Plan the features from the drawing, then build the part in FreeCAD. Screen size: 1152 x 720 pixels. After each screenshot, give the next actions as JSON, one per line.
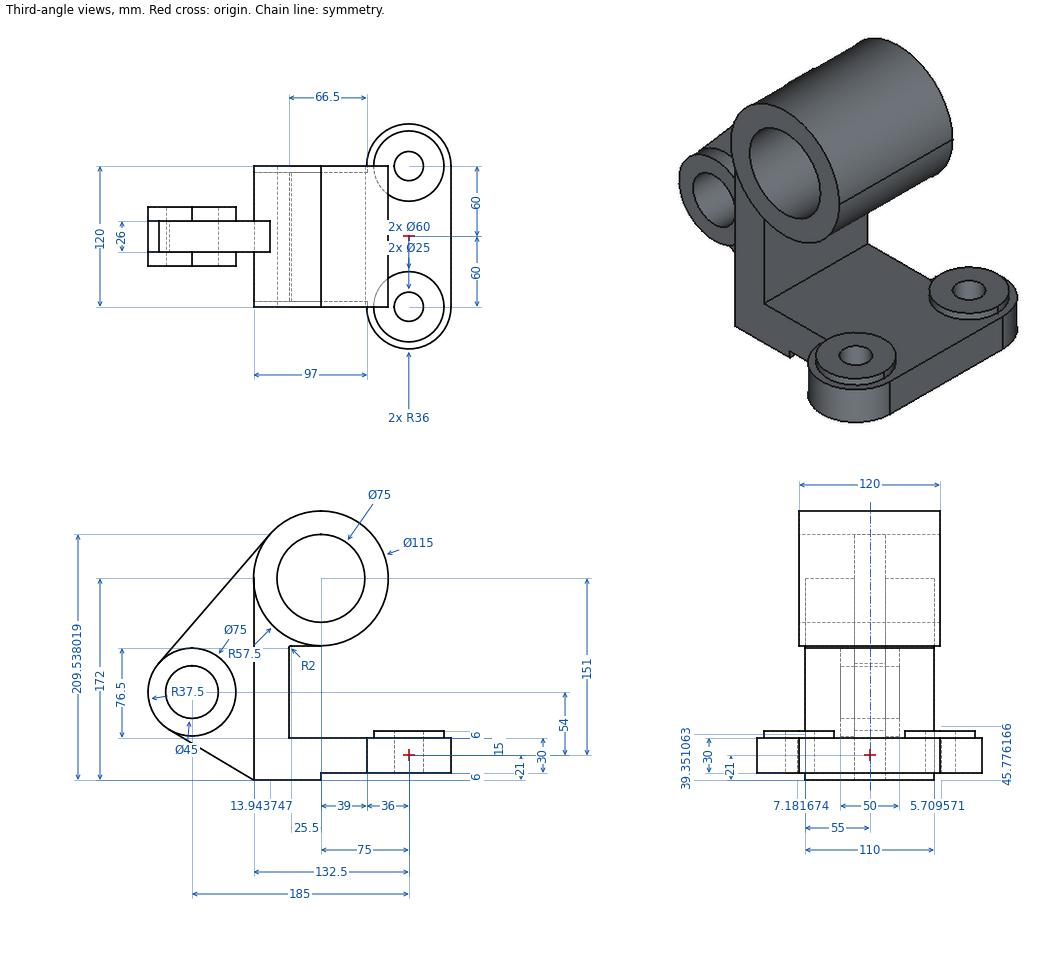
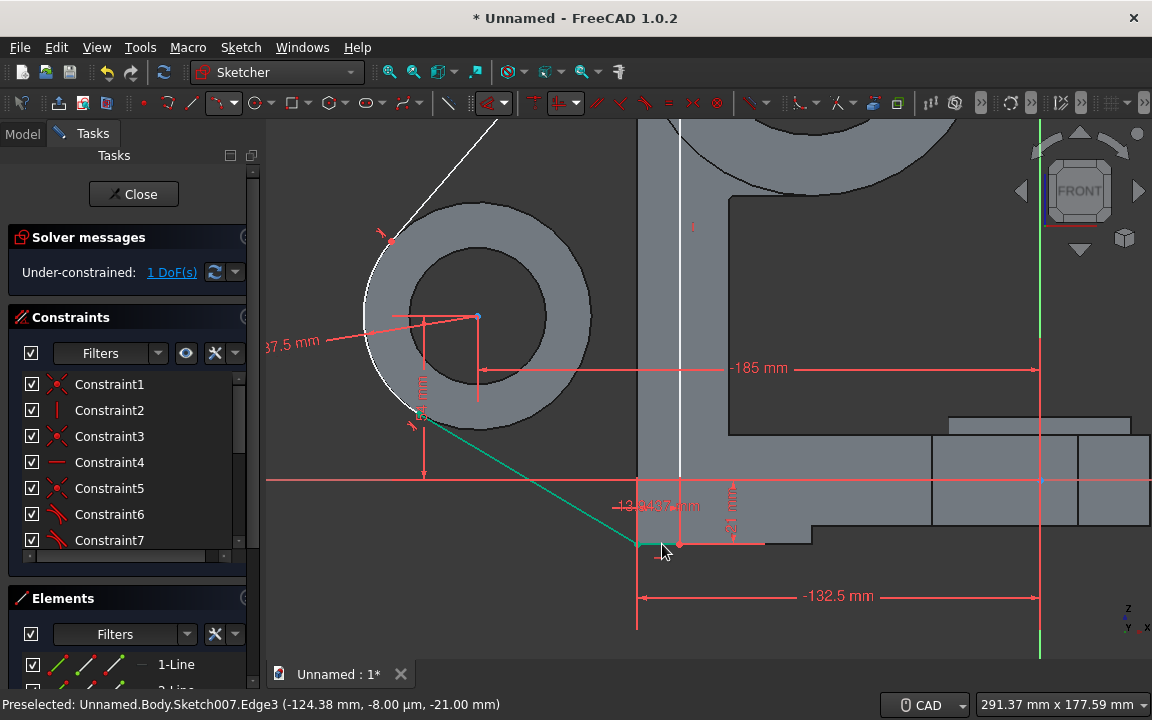
{"action": "left_click", "coordinate": [680, 353]}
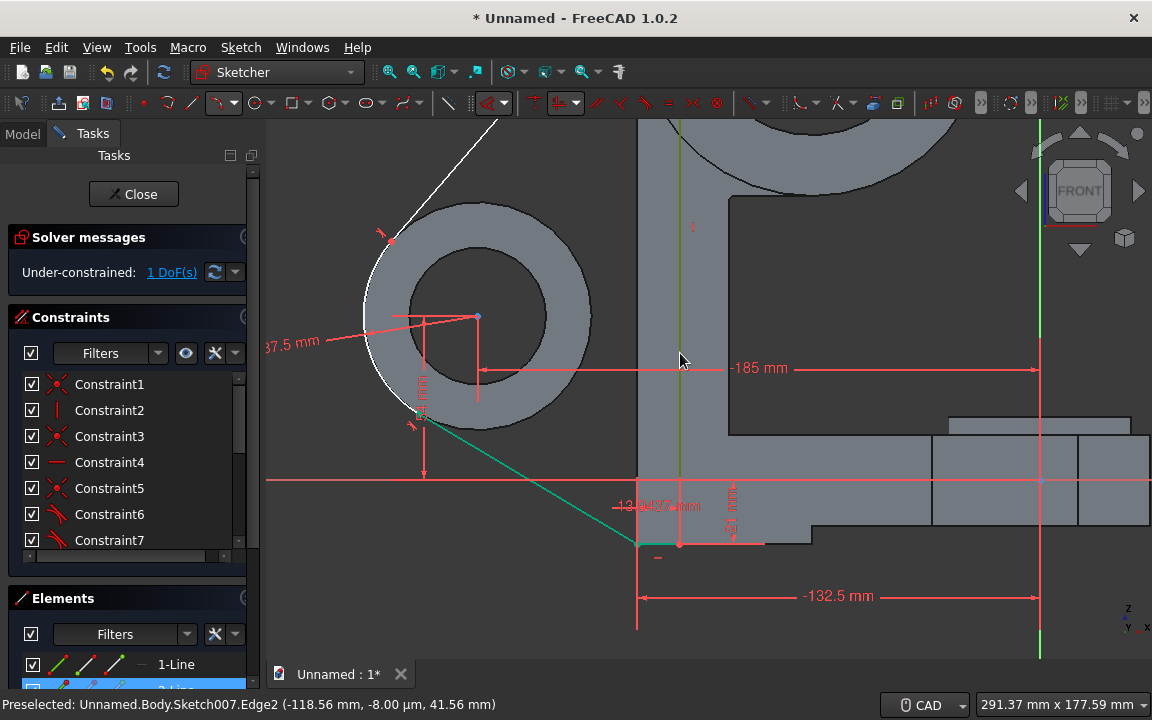
{"action": "key", "text": "i"}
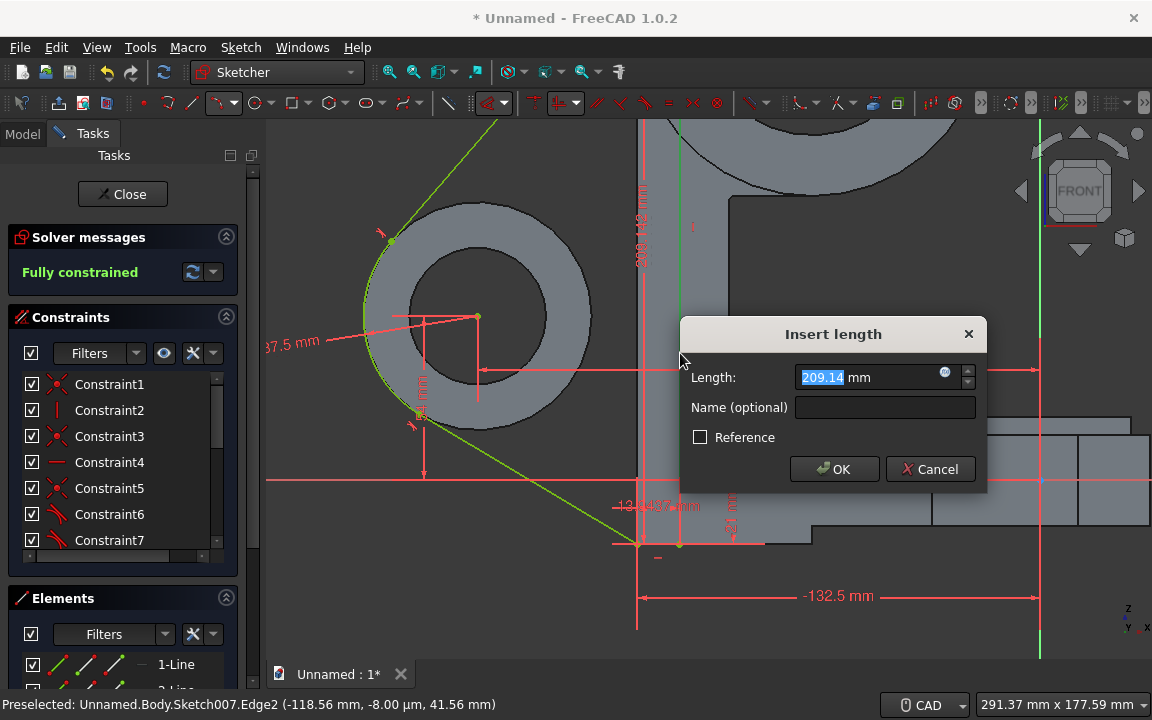
{"action": "type", "text": "209.538019"}
{"action": "key", "text": "Return"}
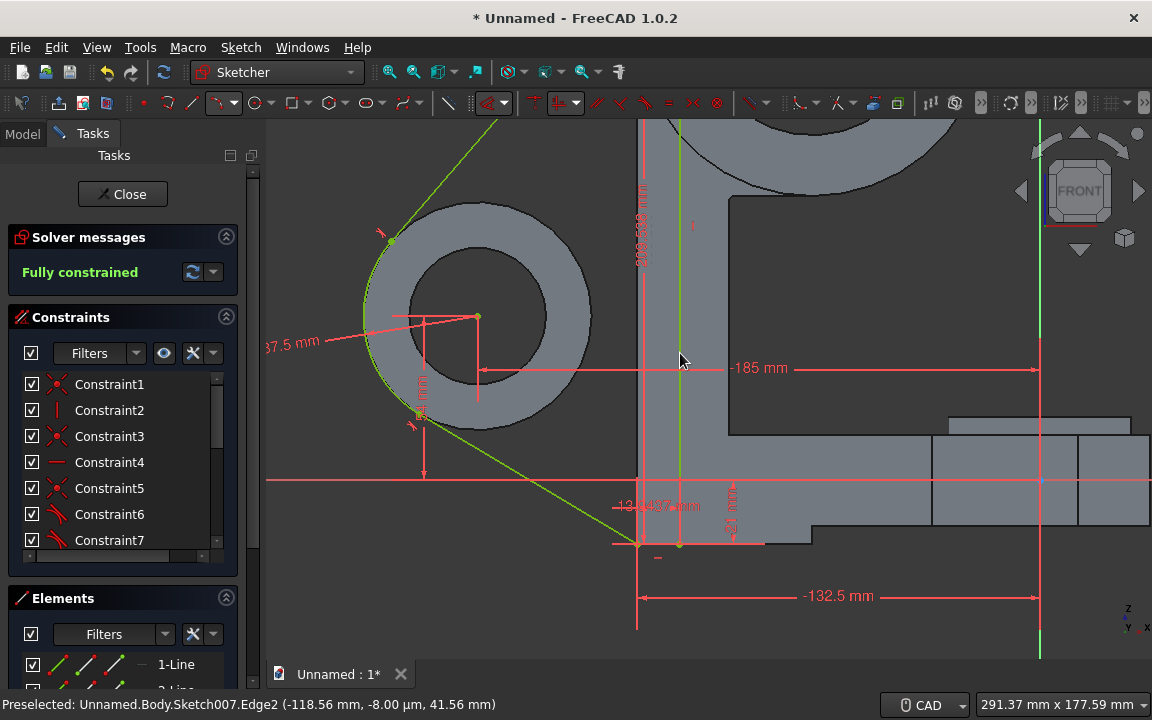
{"action": "left_click", "coordinate": [123, 194]}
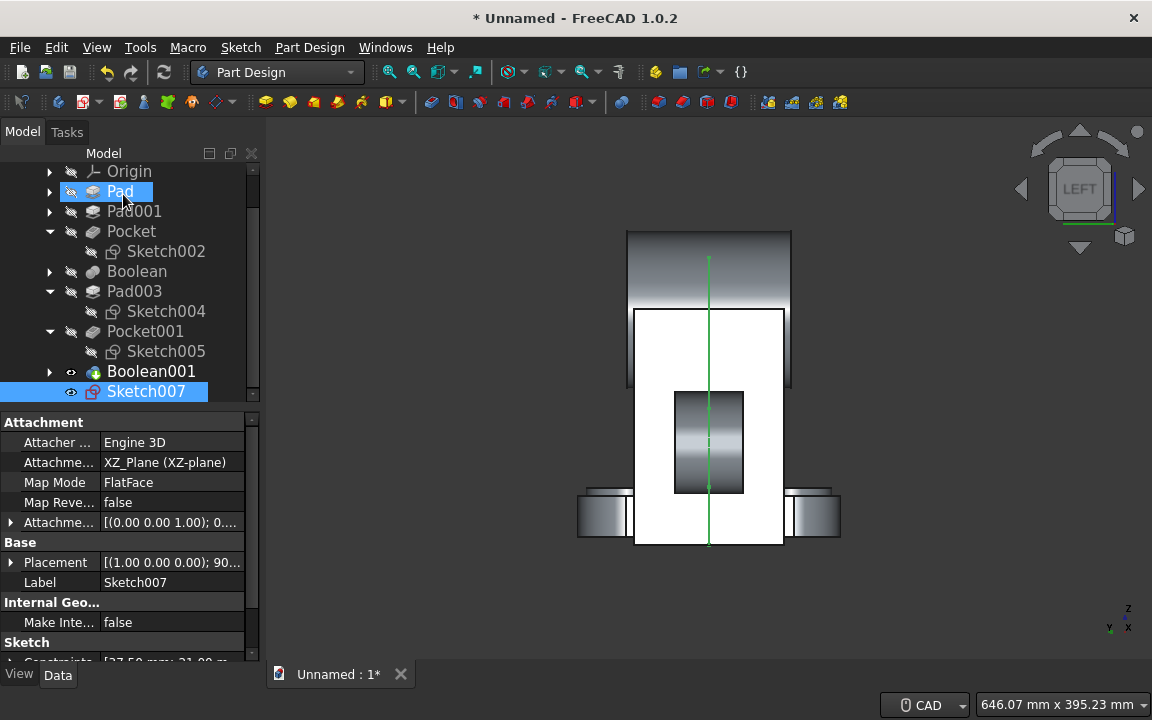
{"action": "left_click", "coordinate": [266, 102]}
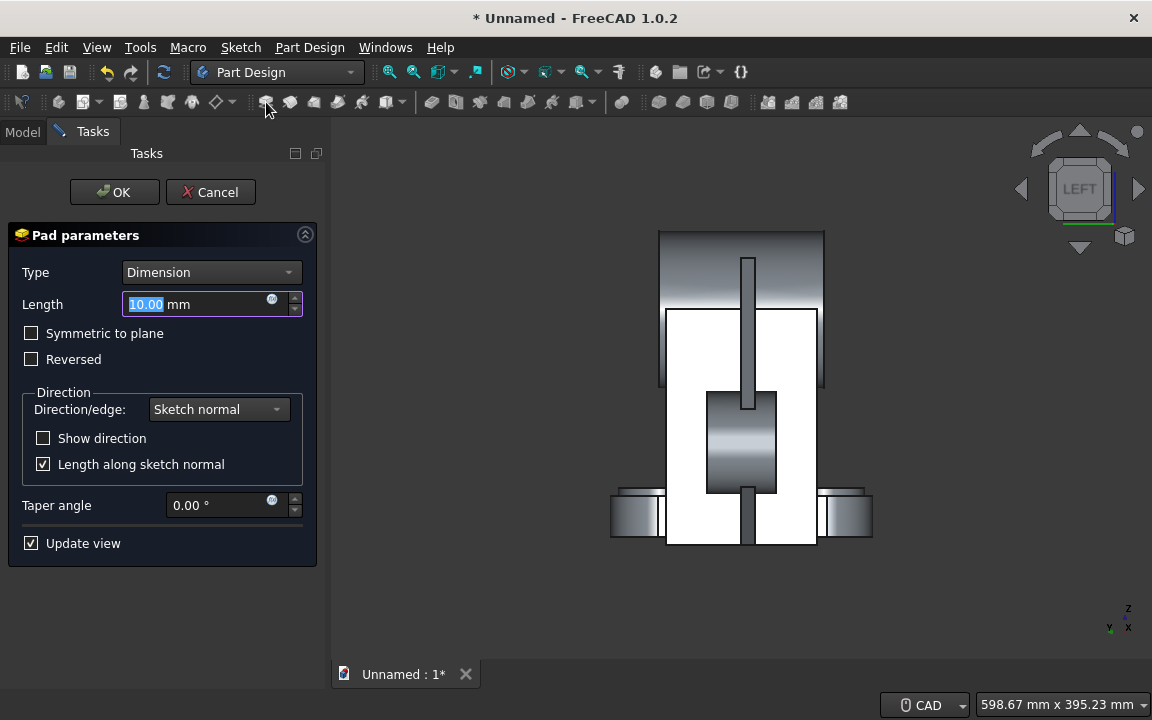
{"action": "type", "text": "26"}
{"action": "key", "text": "Tab"}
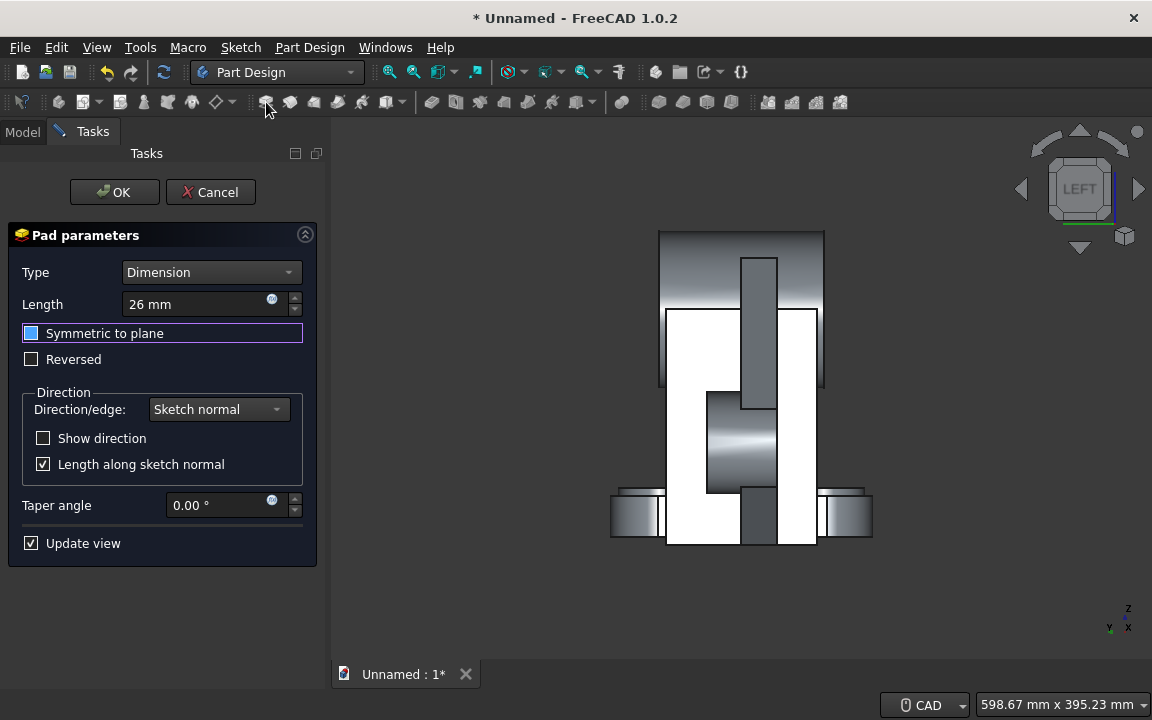
{"action": "left_click", "coordinate": [30, 333]}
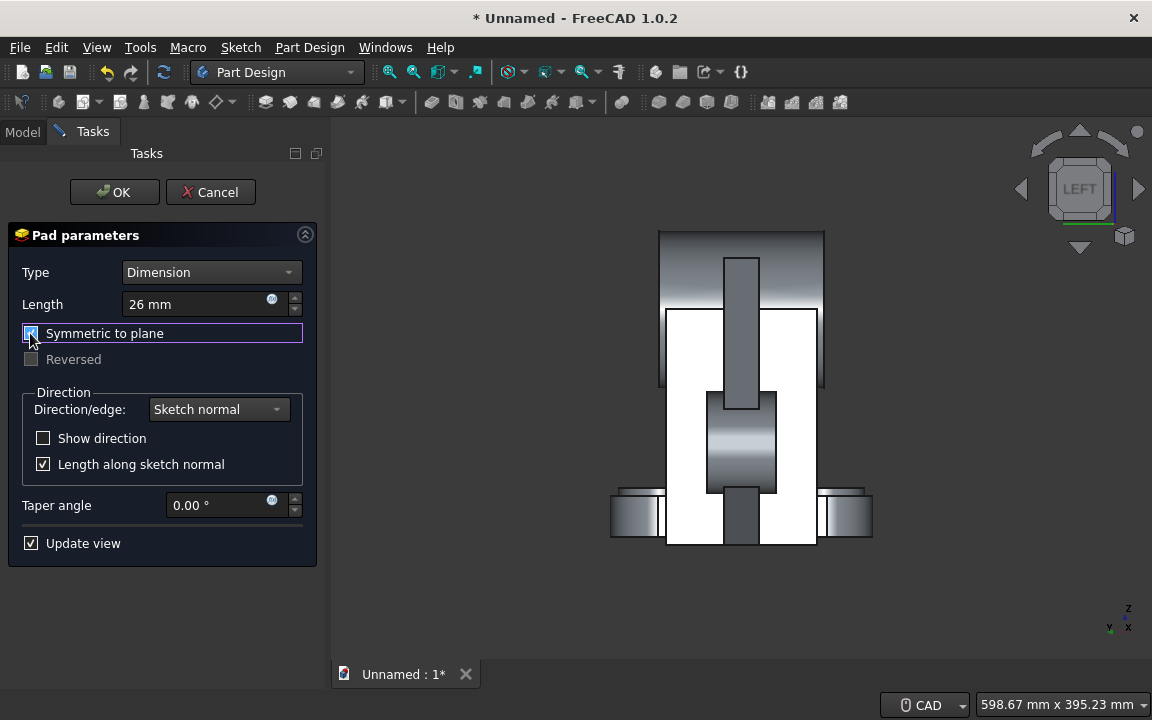
{"action": "left_click", "coordinate": [115, 192]}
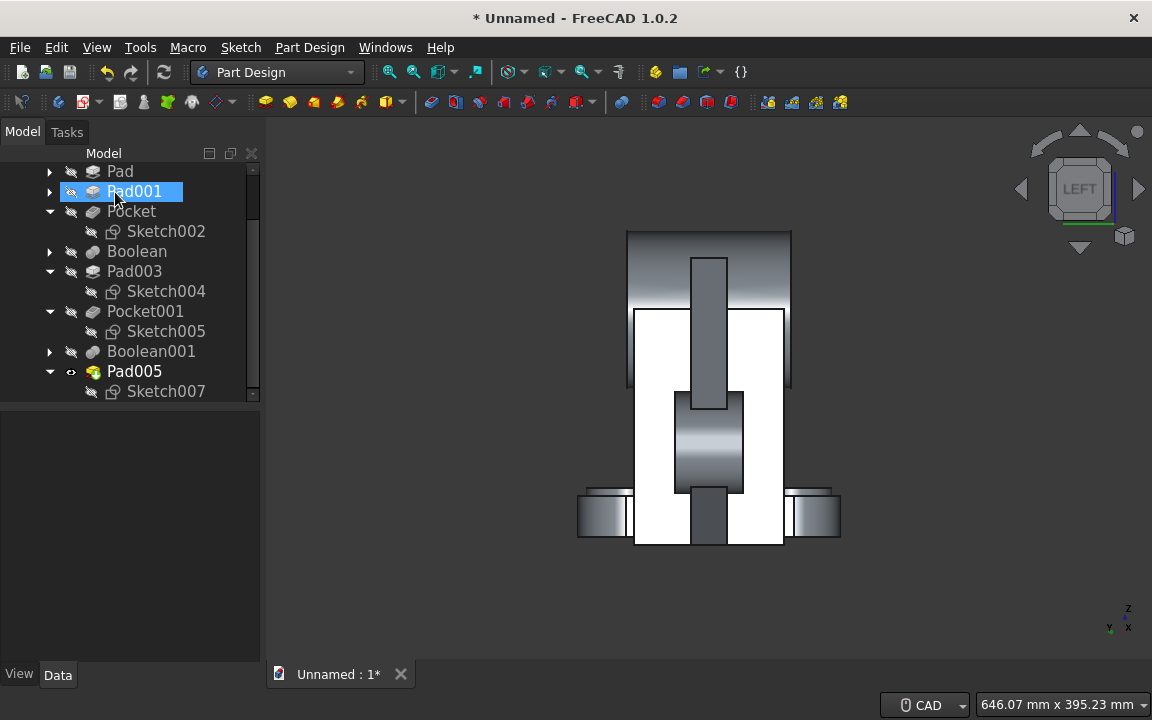
{"action": "key", "text": "0"}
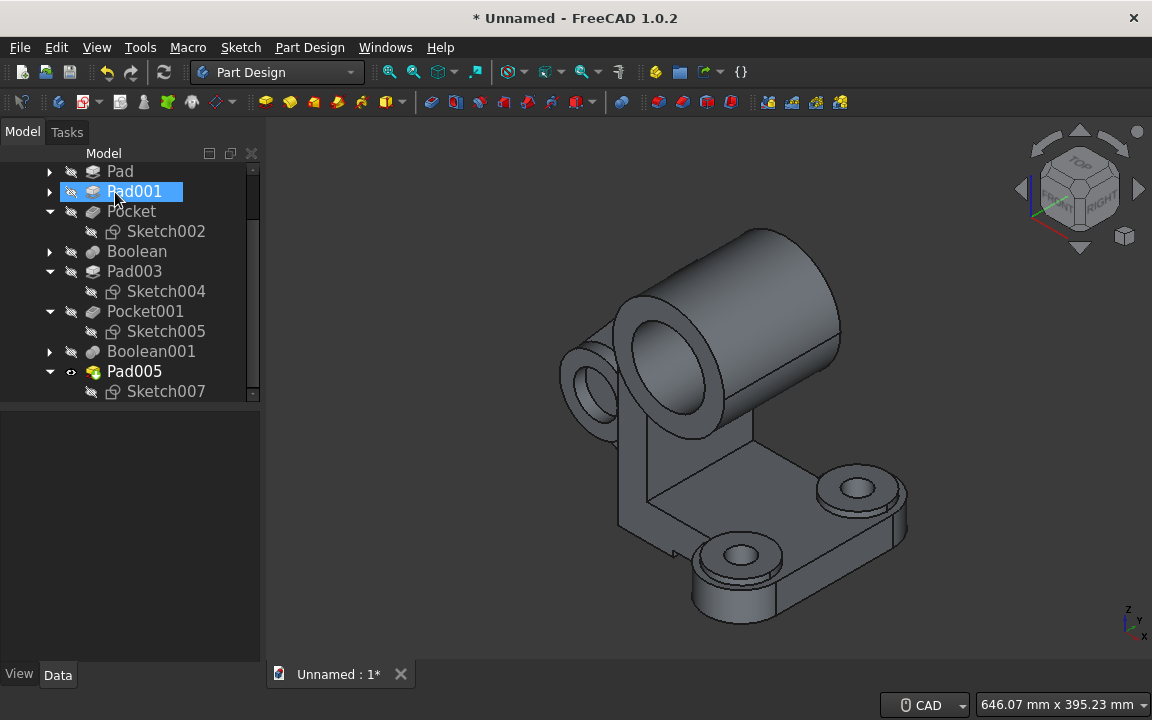
{"action": "left_click", "coordinate": [575, 358]}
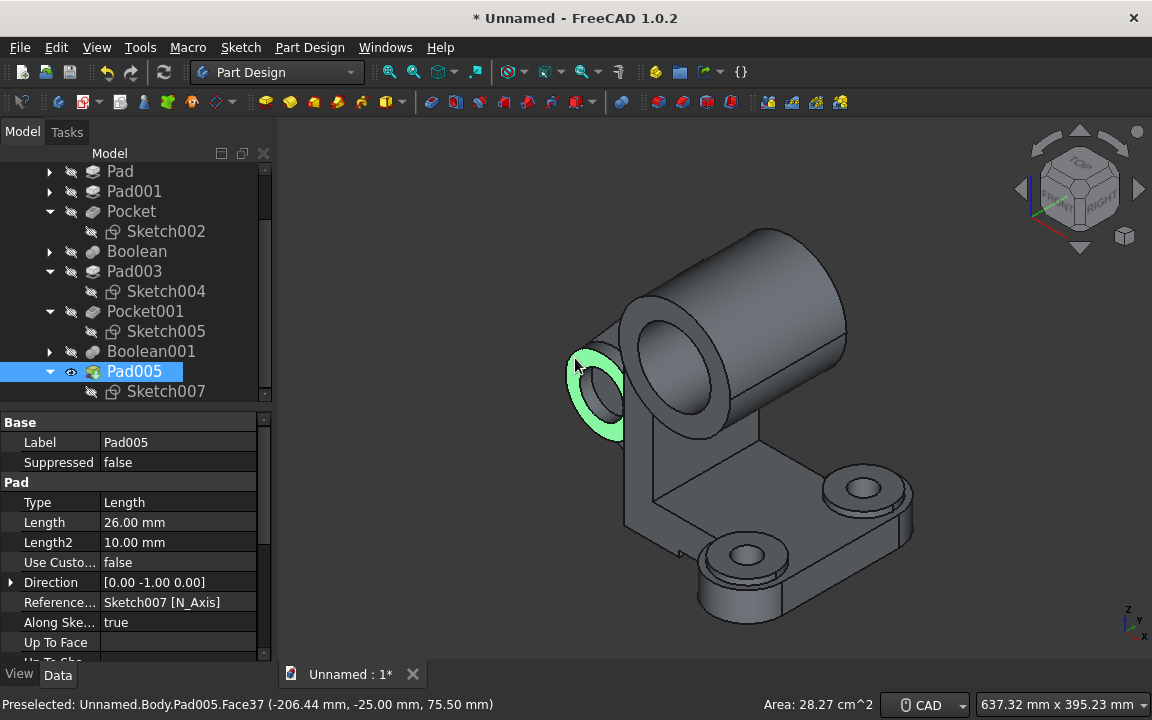
{"action": "left_click", "coordinate": [84, 102]}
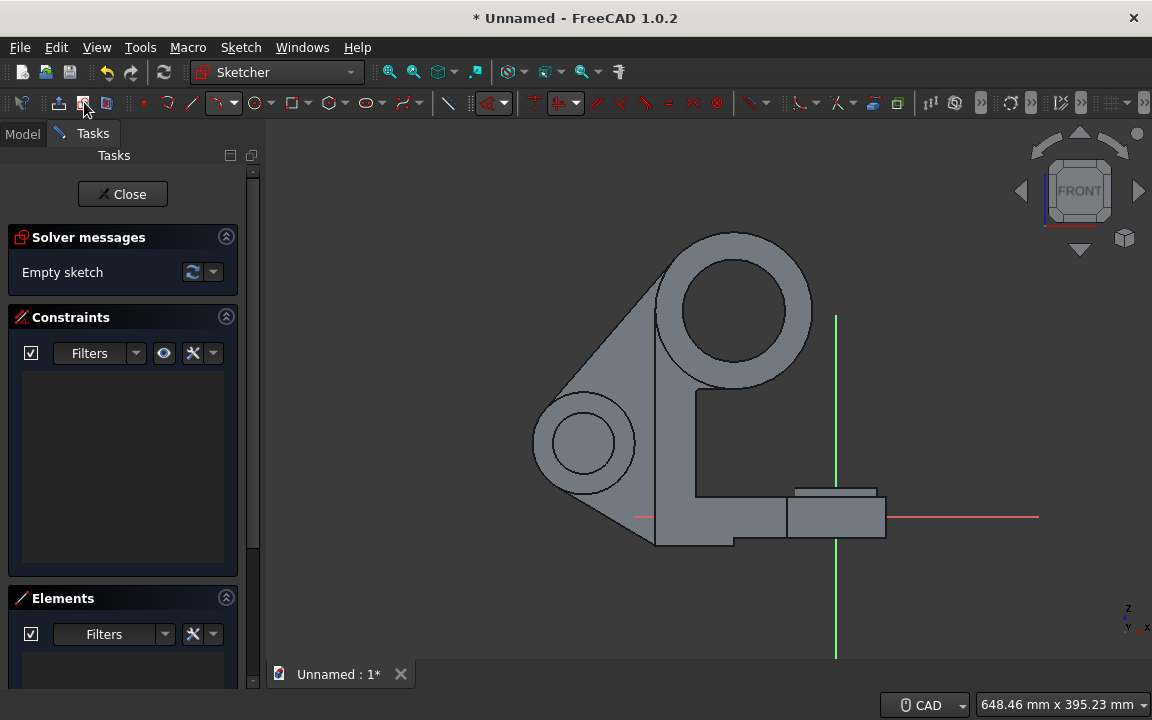
{"action": "left_click", "coordinate": [108, 104]}